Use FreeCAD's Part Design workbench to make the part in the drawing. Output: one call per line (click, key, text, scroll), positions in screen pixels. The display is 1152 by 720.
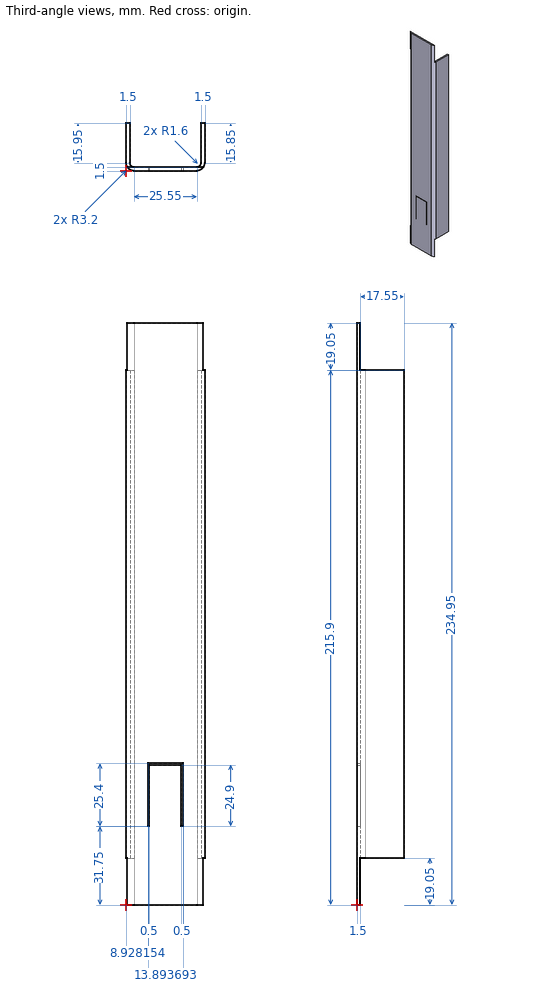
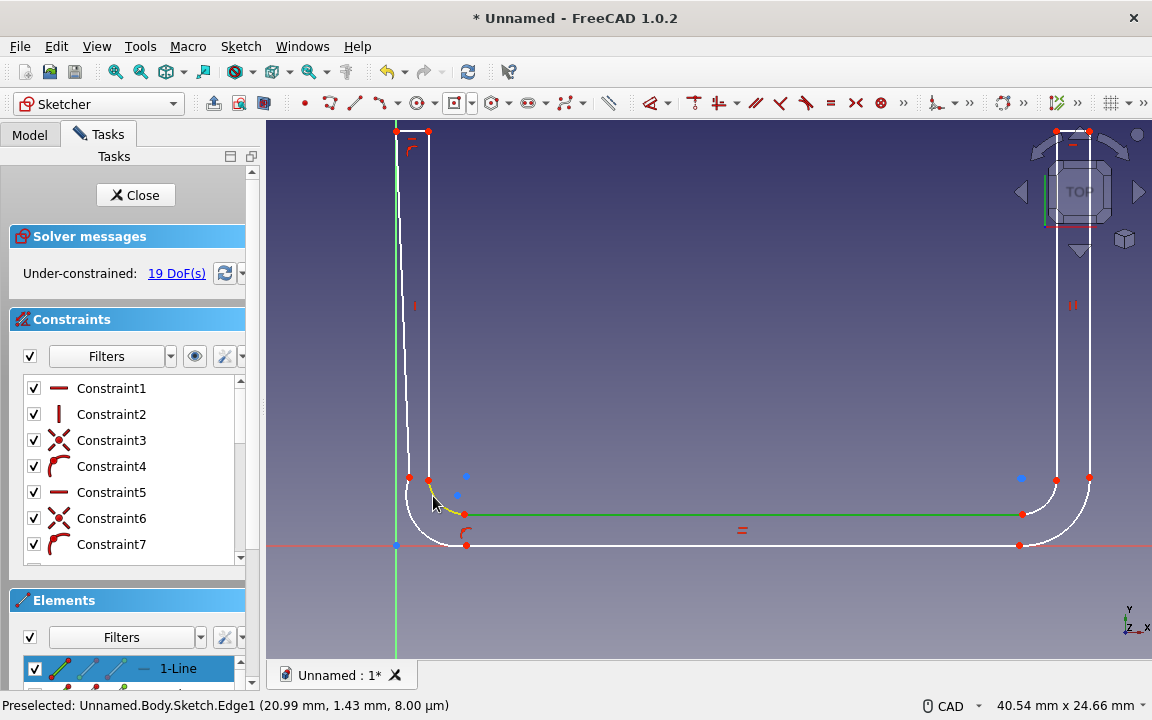
click(434, 496)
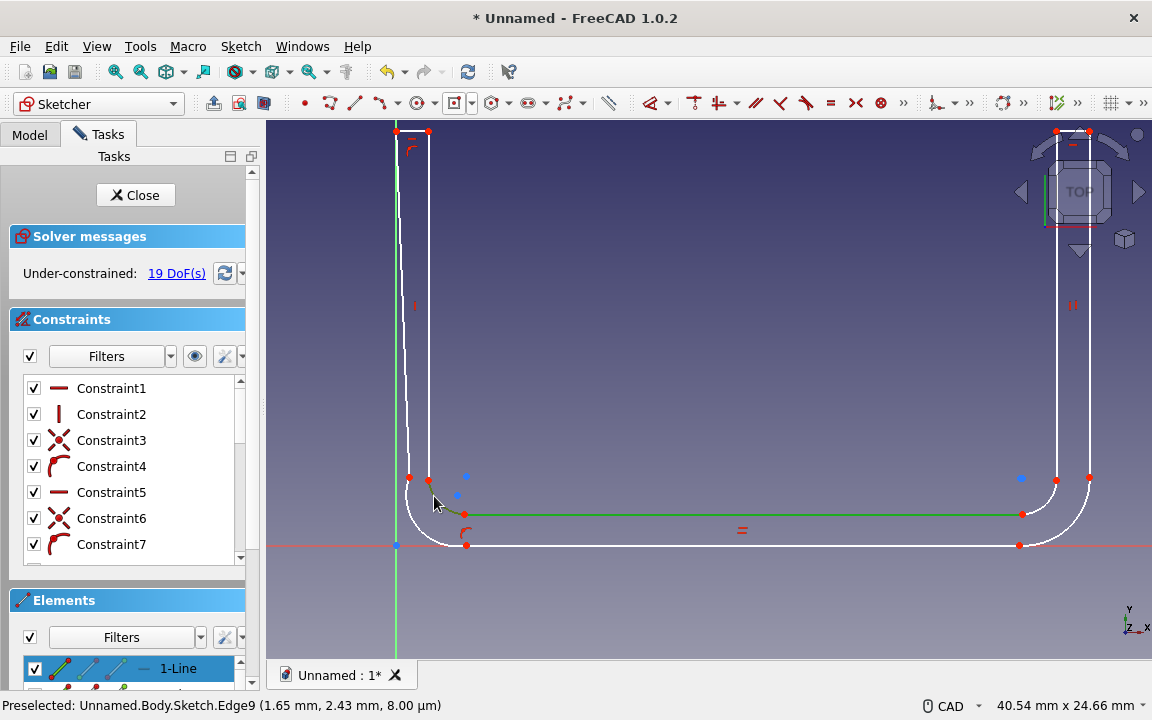
click(806, 104)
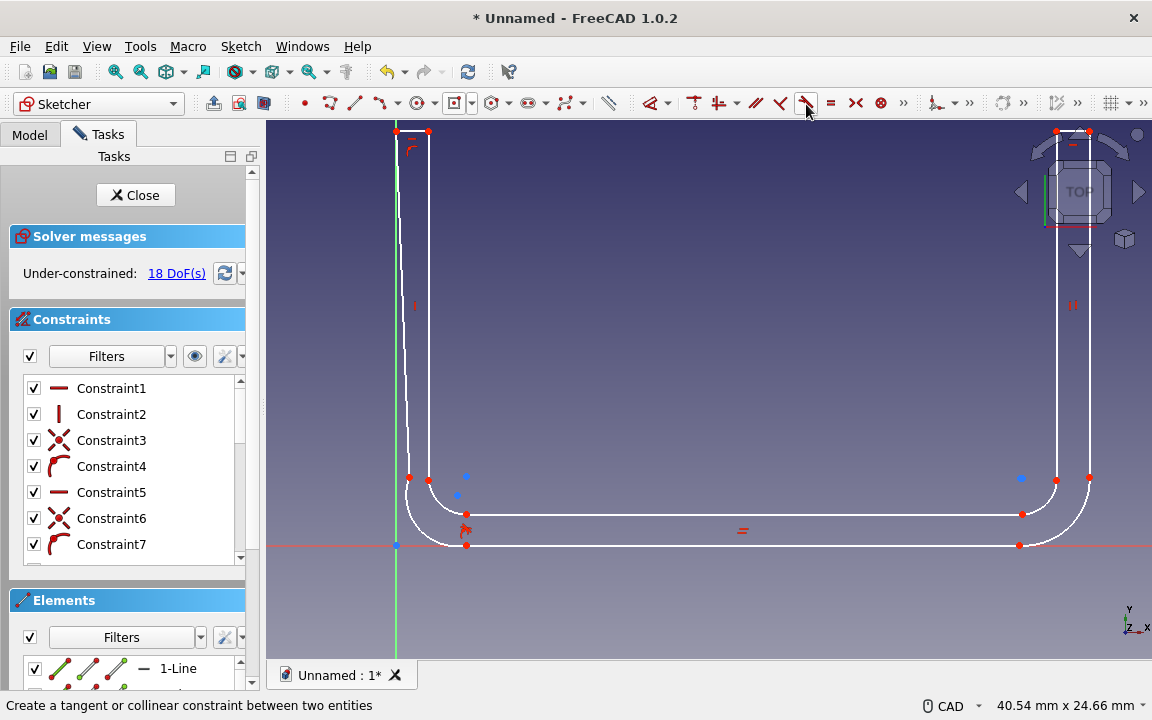
click(856, 515)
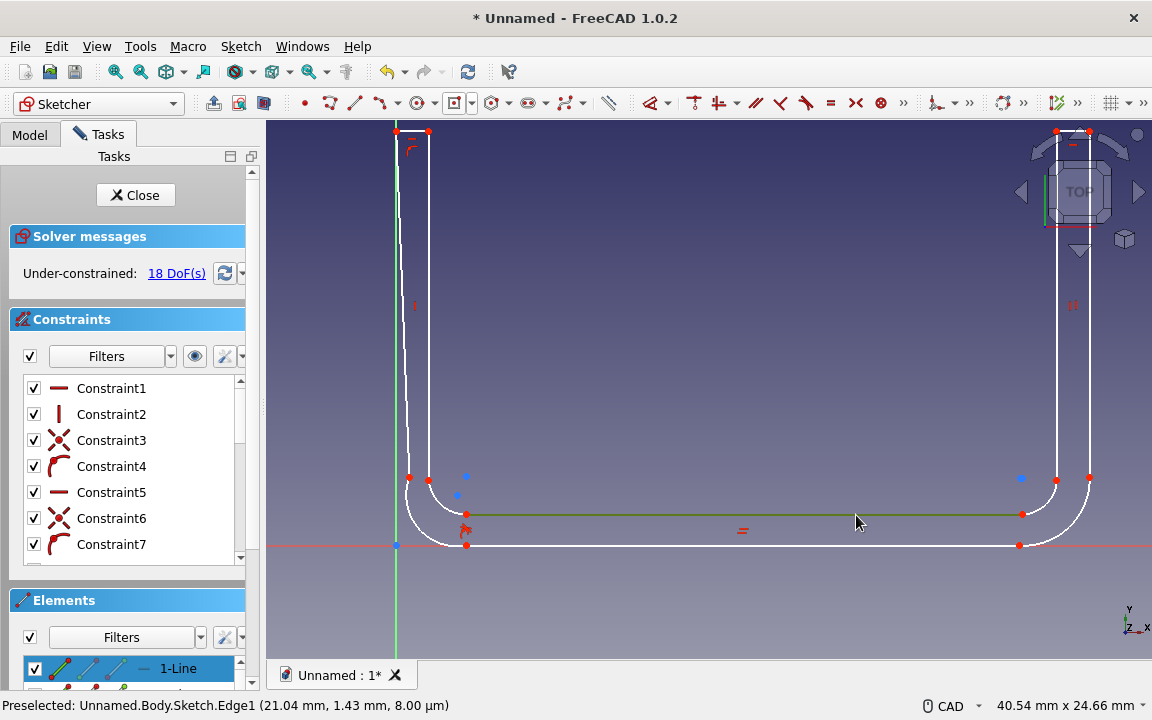
scroll(432, 495, down, 2)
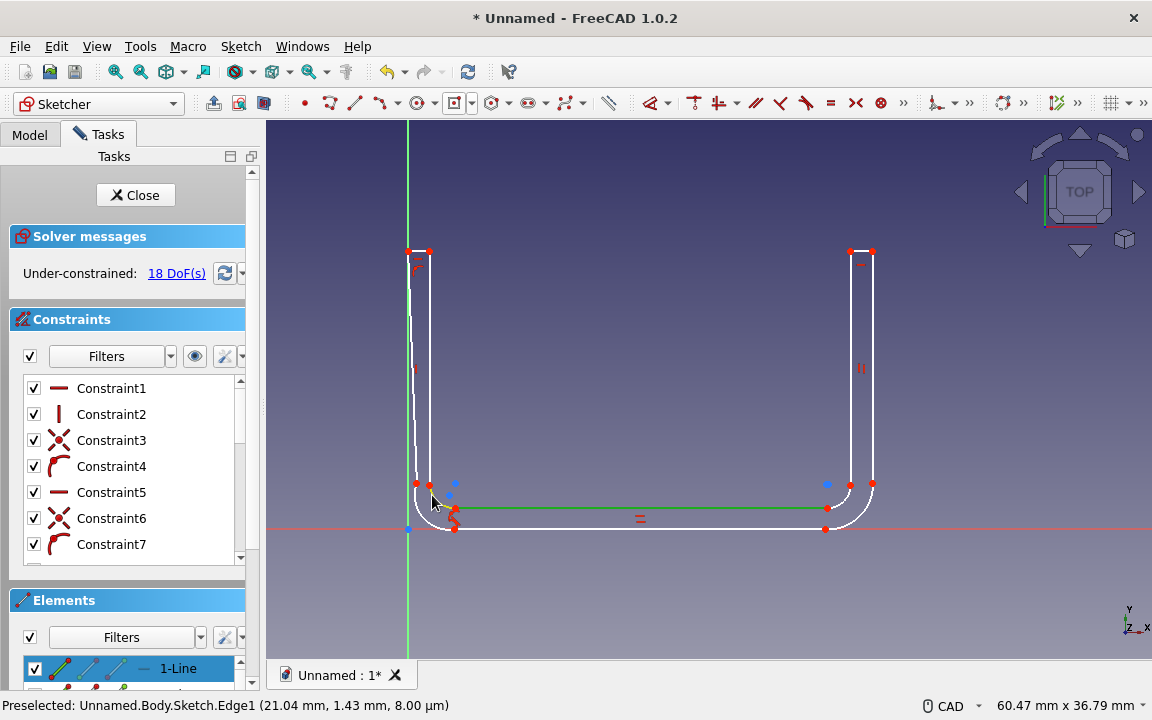
scroll(838, 505, up, 2)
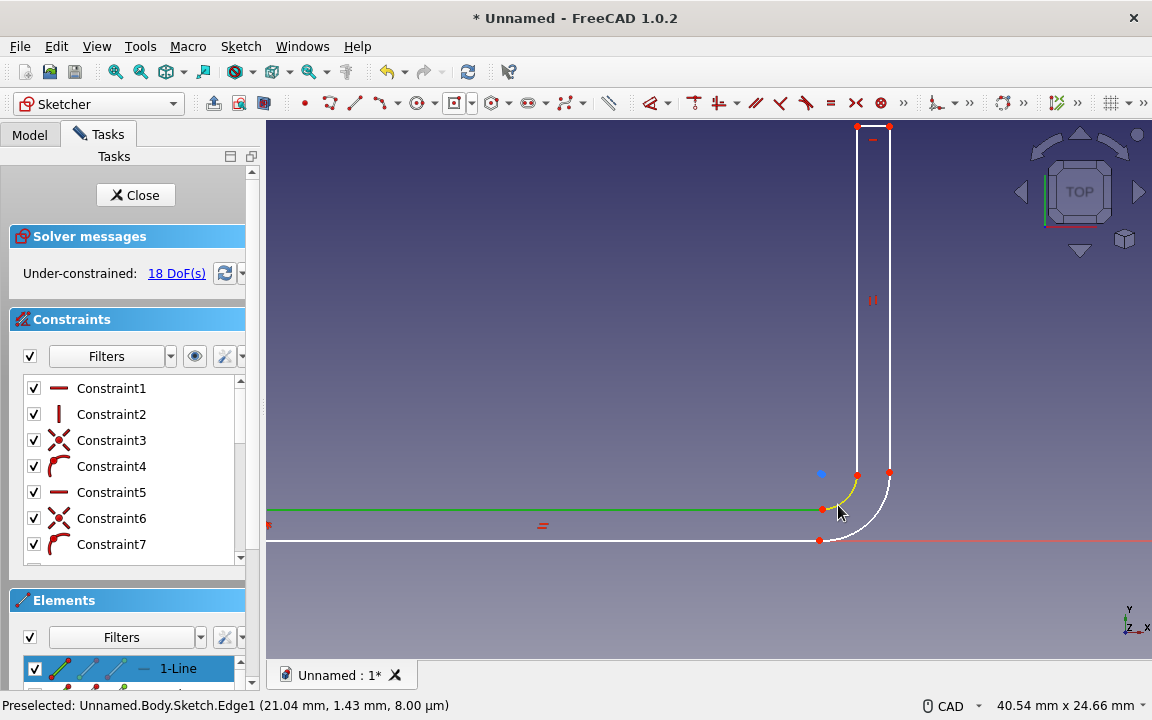
click(838, 505)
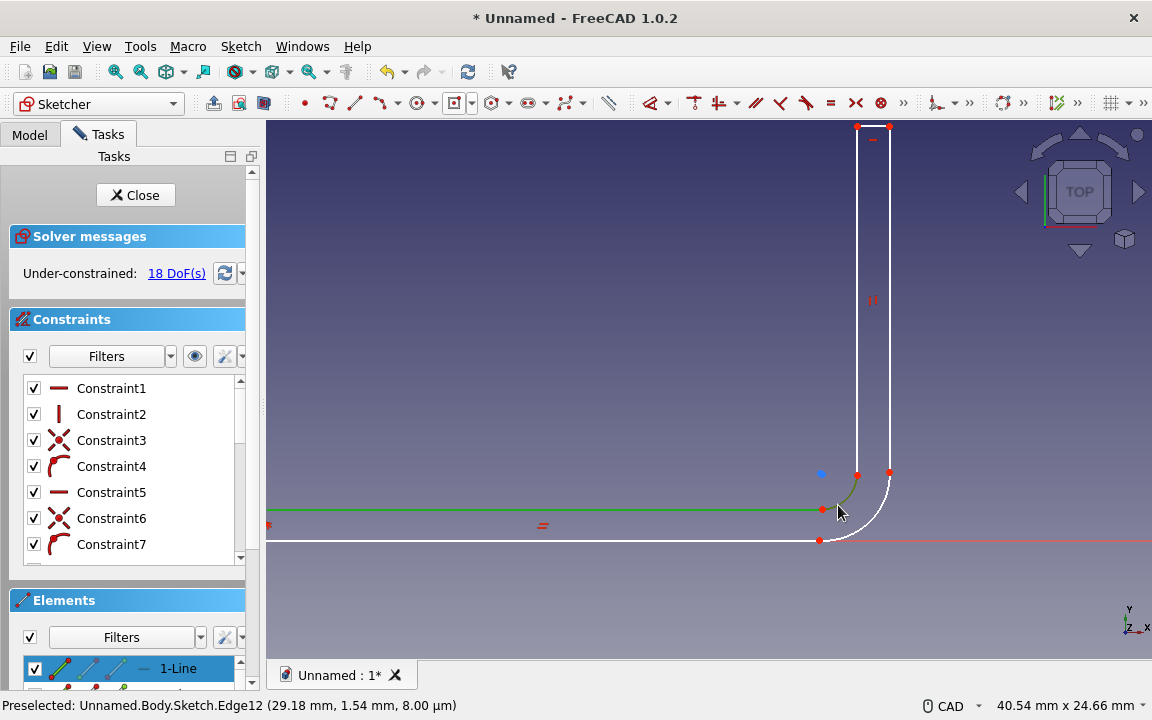
click(806, 104)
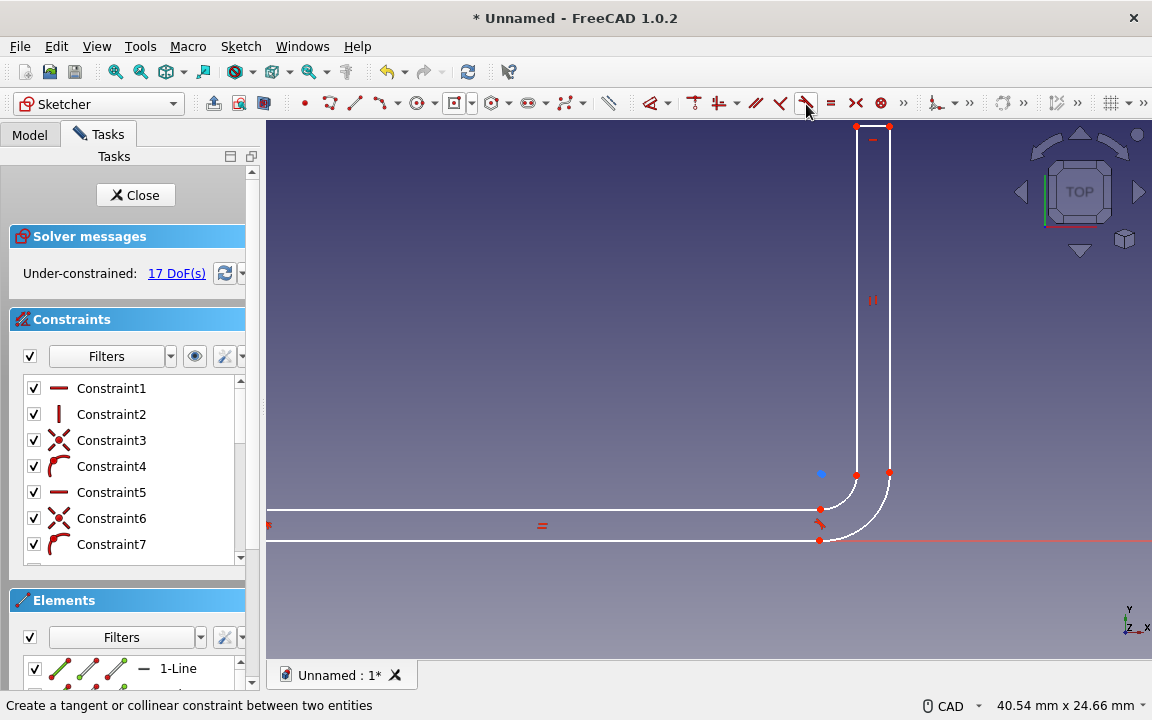
scroll(838, 505, down, 2)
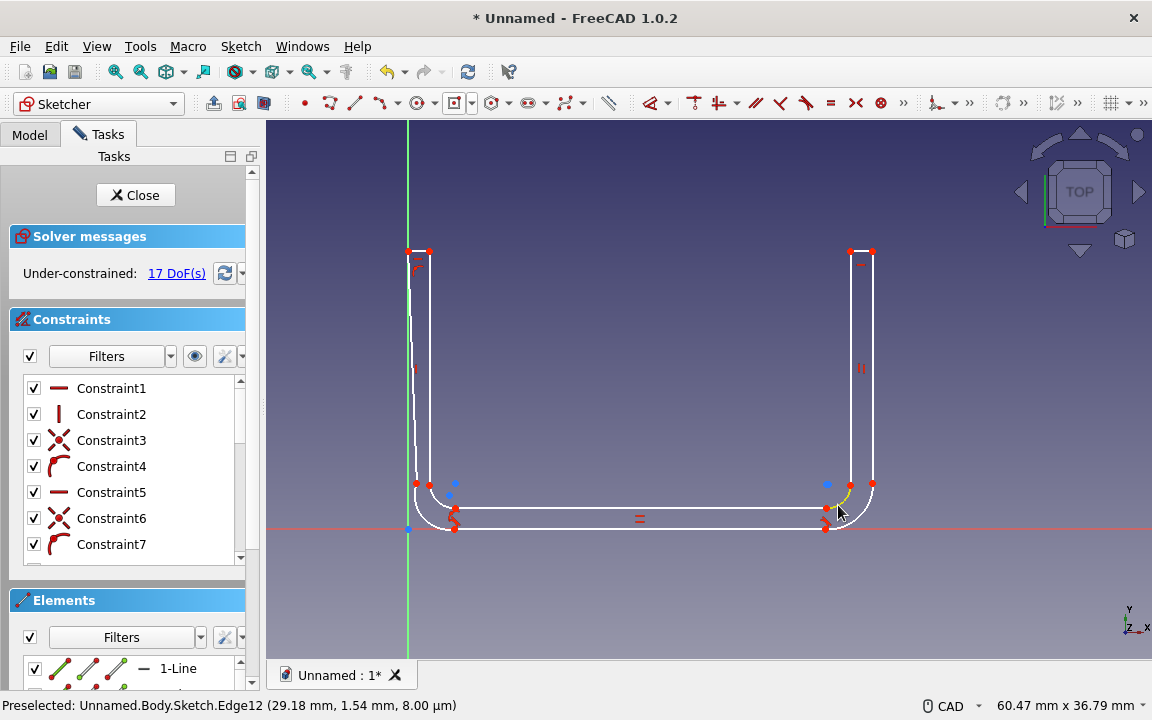
click(430, 415)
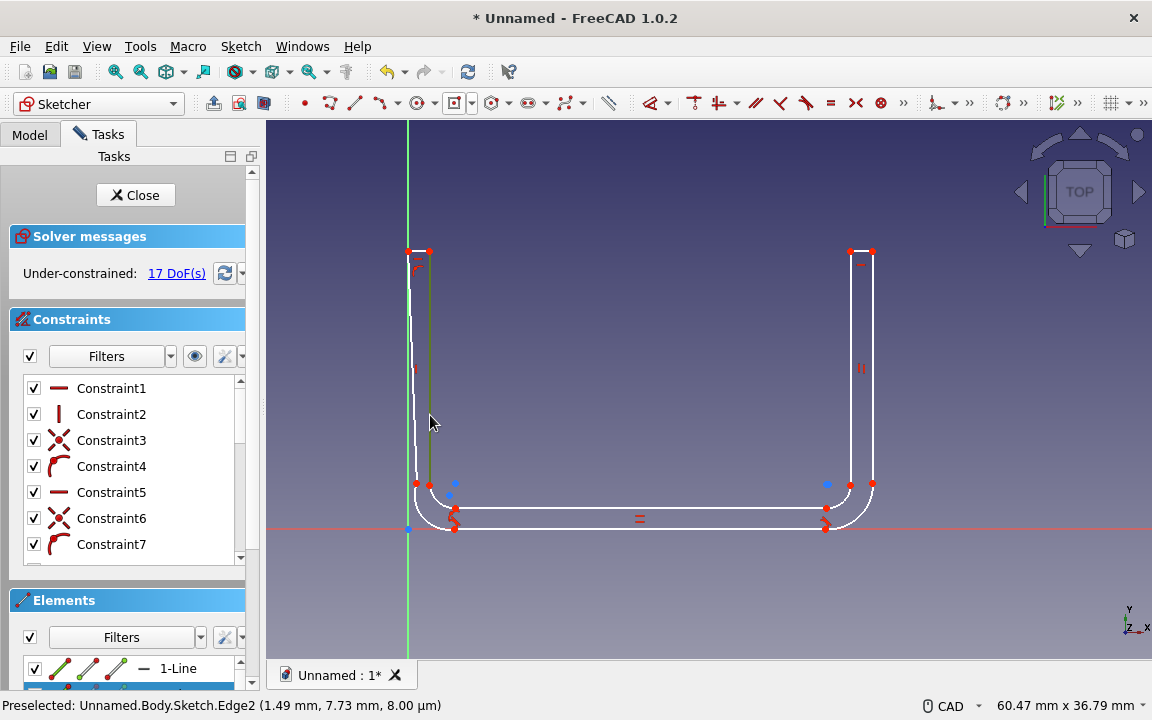
scroll(433, 496, up, 2)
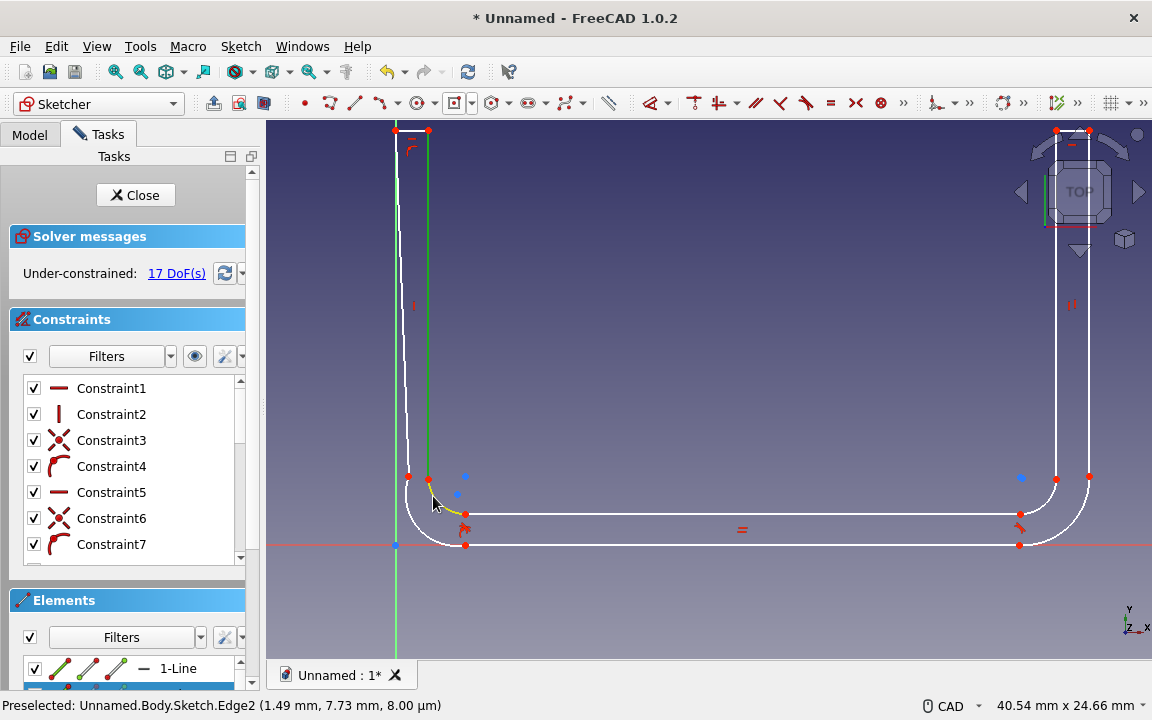
click(433, 496)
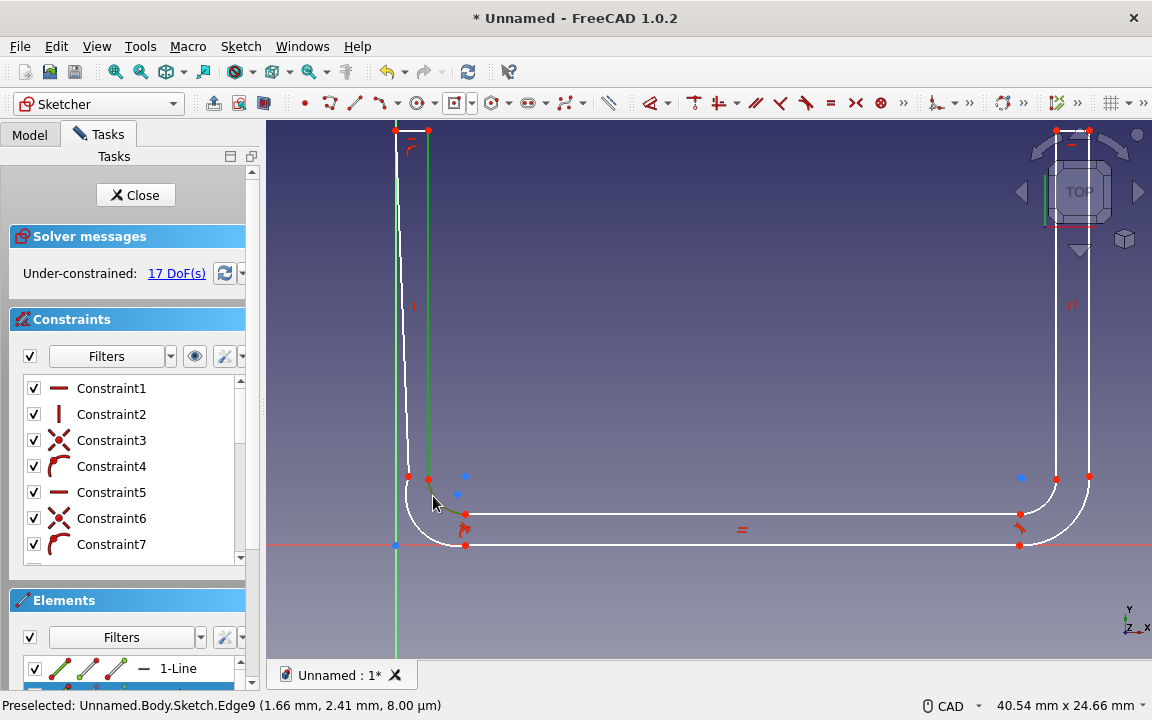
click(806, 104)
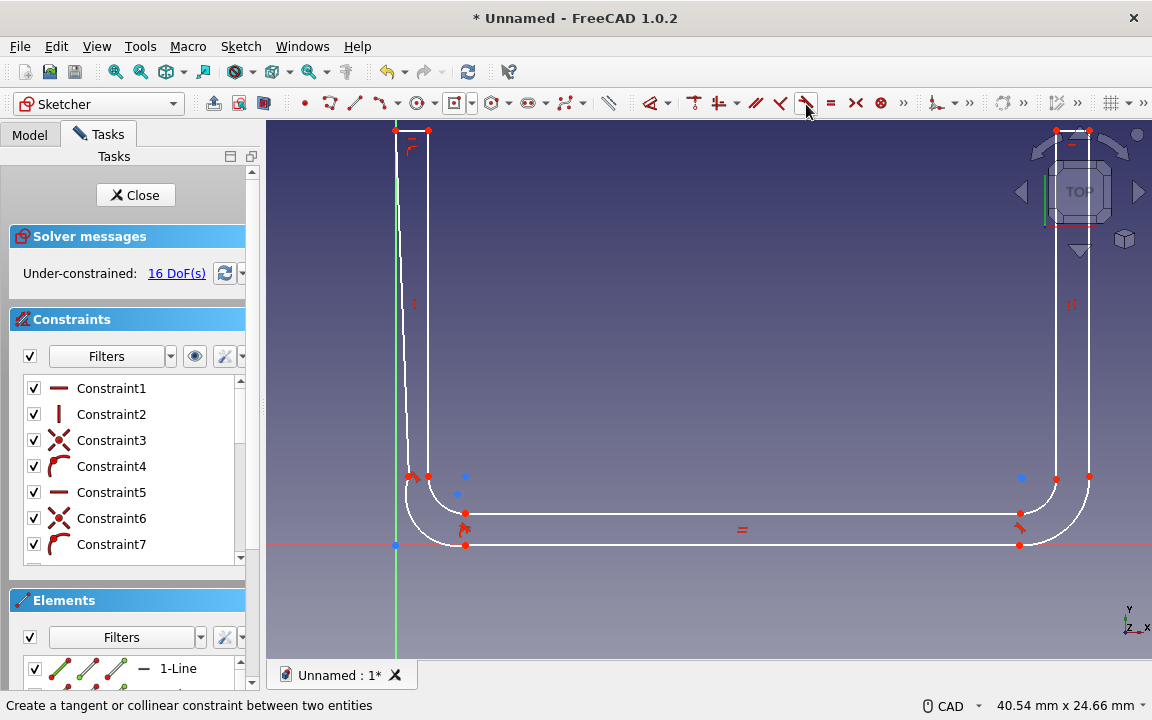
click(400, 234)